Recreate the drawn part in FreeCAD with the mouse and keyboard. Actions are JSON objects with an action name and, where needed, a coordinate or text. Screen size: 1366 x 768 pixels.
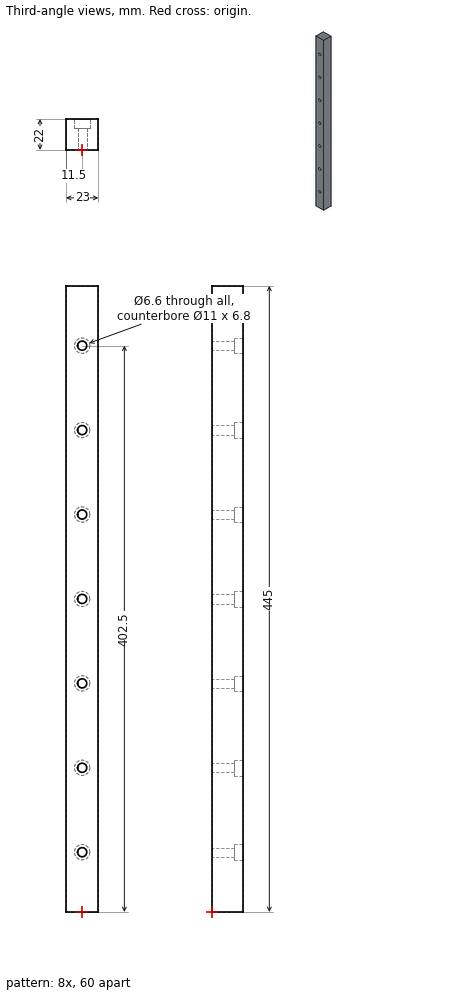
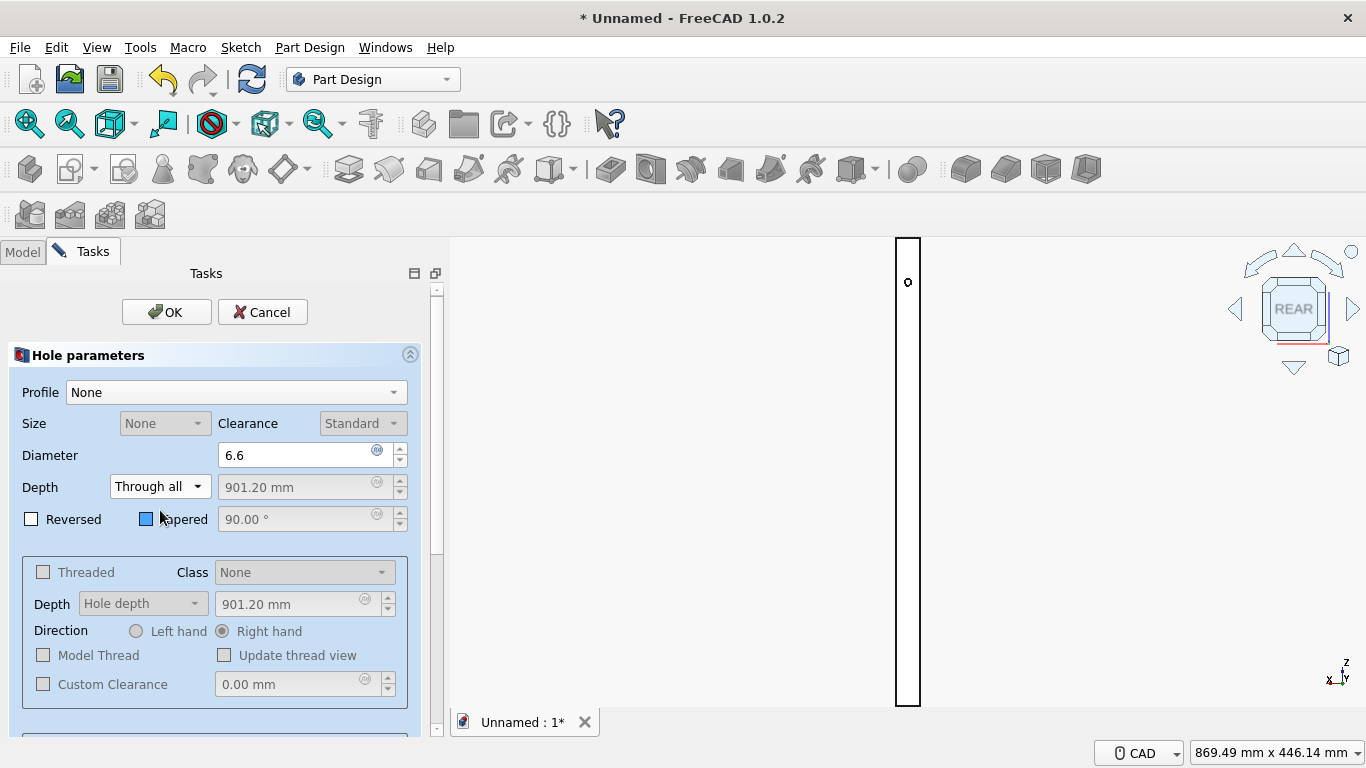
{"action": "scroll", "coordinate": [437, 510], "scroll_direction": "down", "scroll_amount": 2}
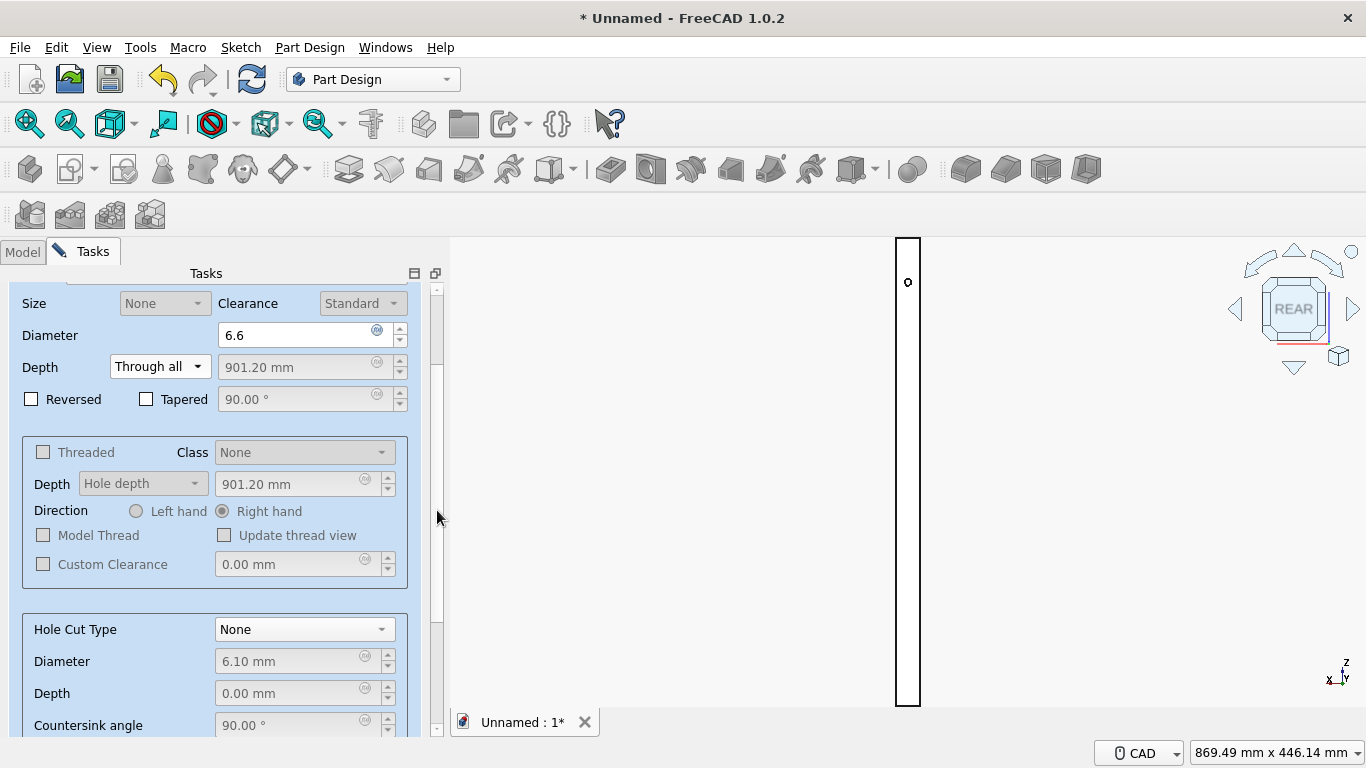
{"action": "left_click", "coordinate": [306, 630]}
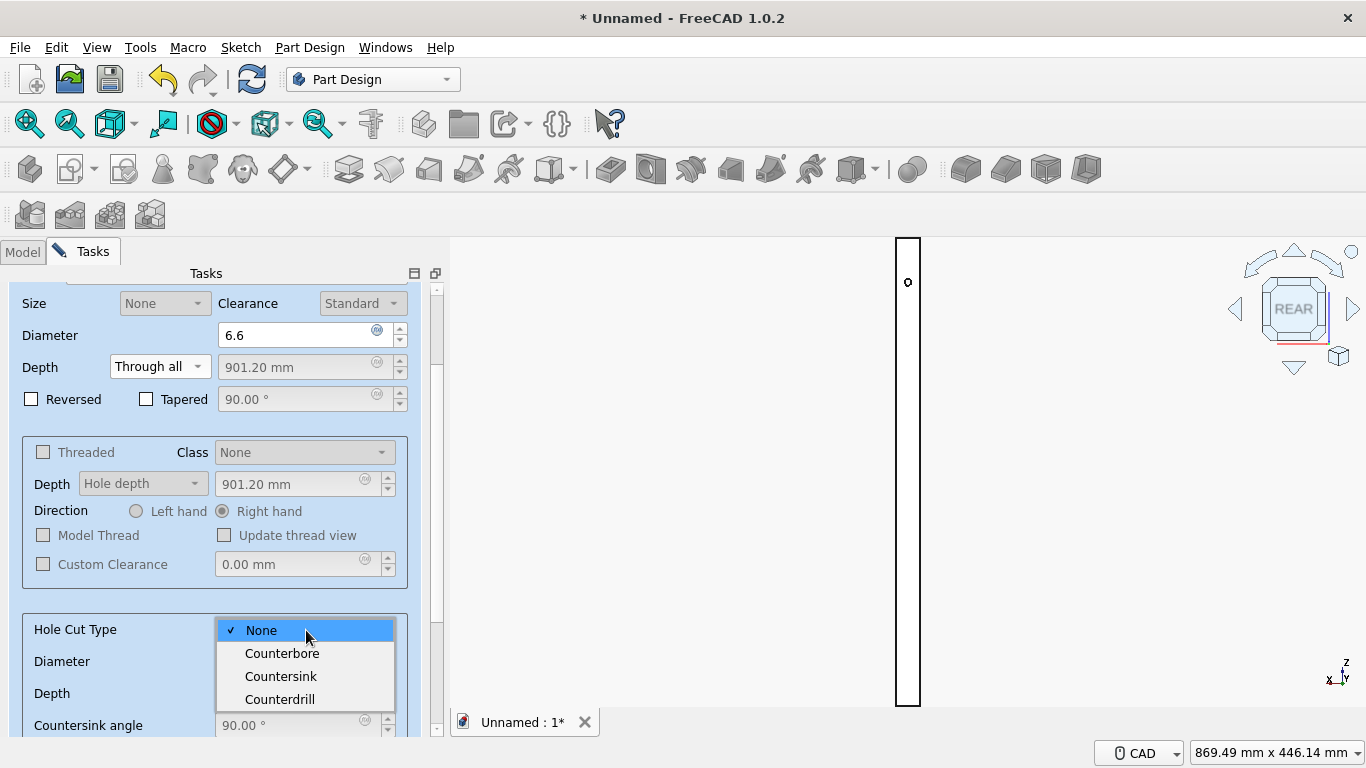
{"action": "left_click", "coordinate": [304, 654]}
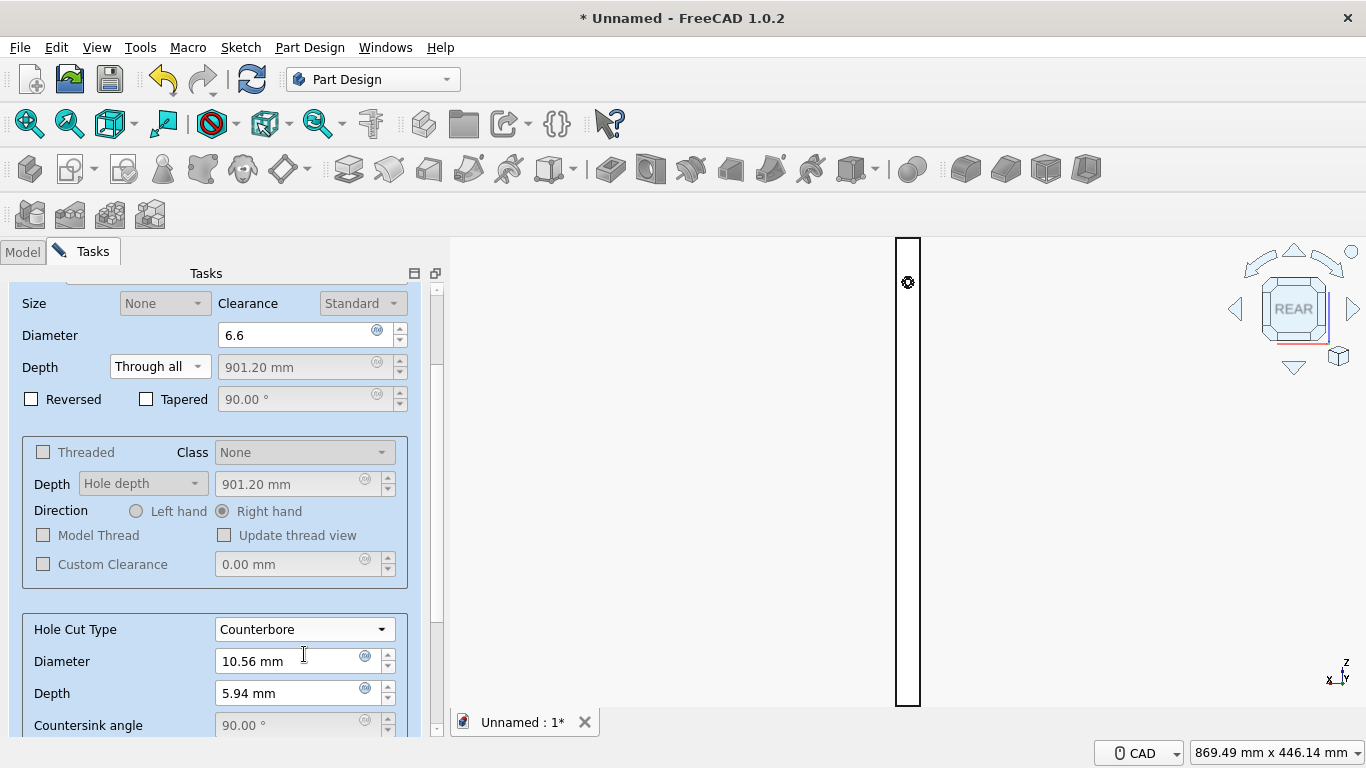
{"action": "triple_click", "coordinate": [298, 661]}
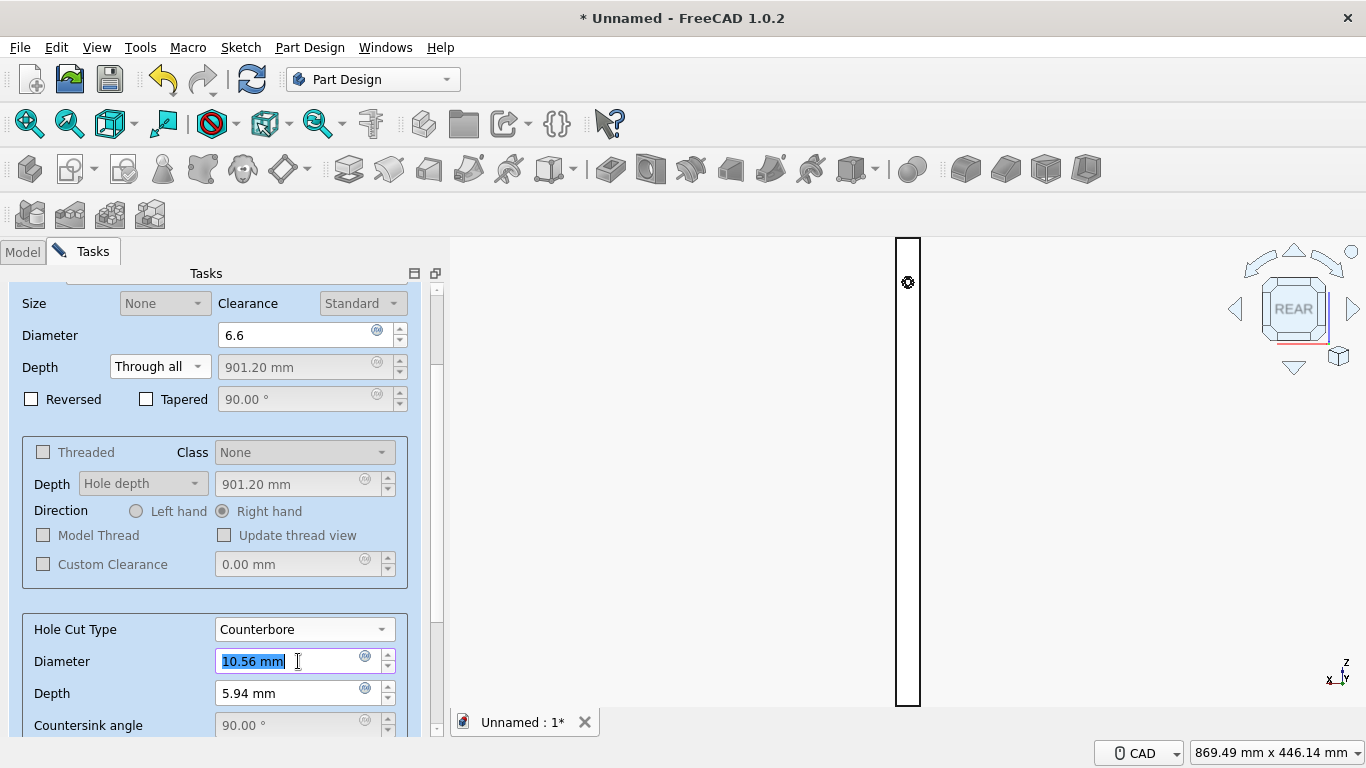
{"action": "type", "text": "11"}
{"action": "key", "text": "Tab"}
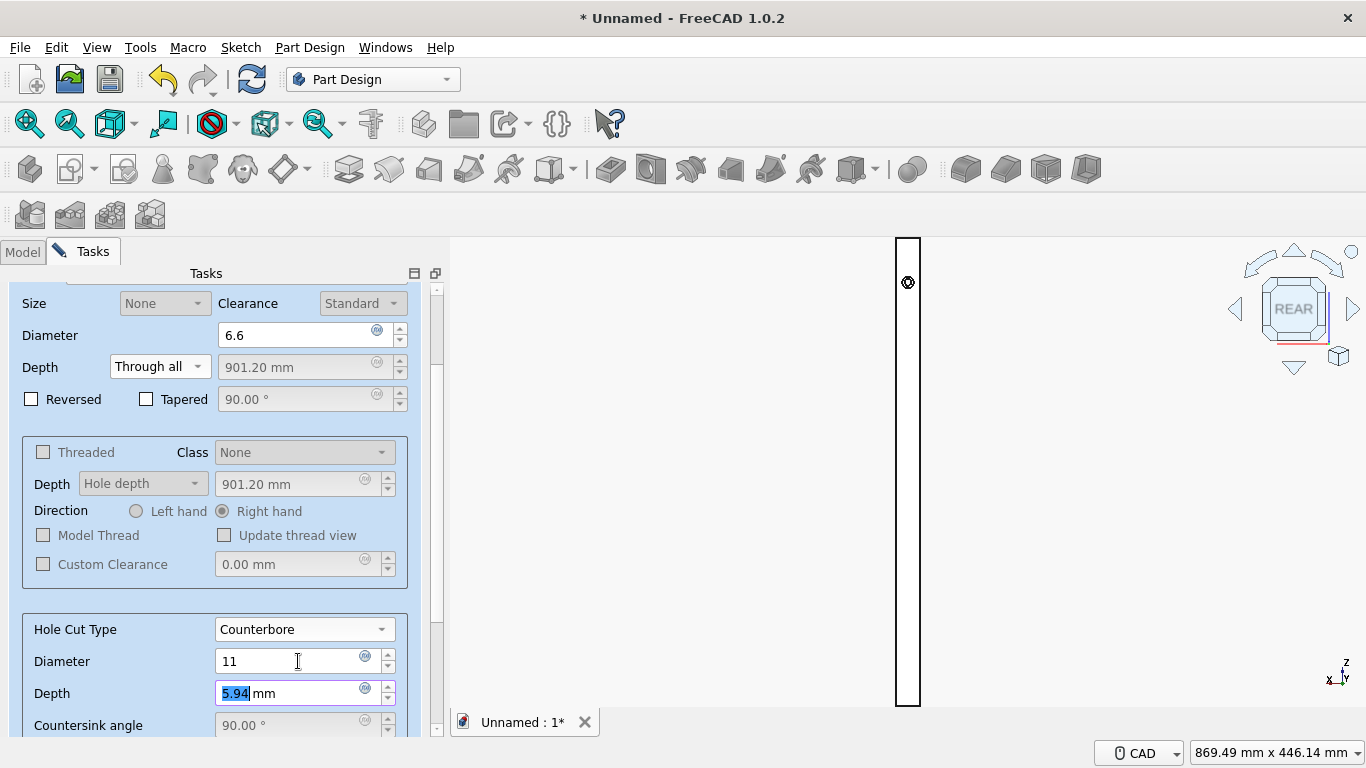
{"action": "type", "text": "6.8"}
{"action": "key", "text": "Tab"}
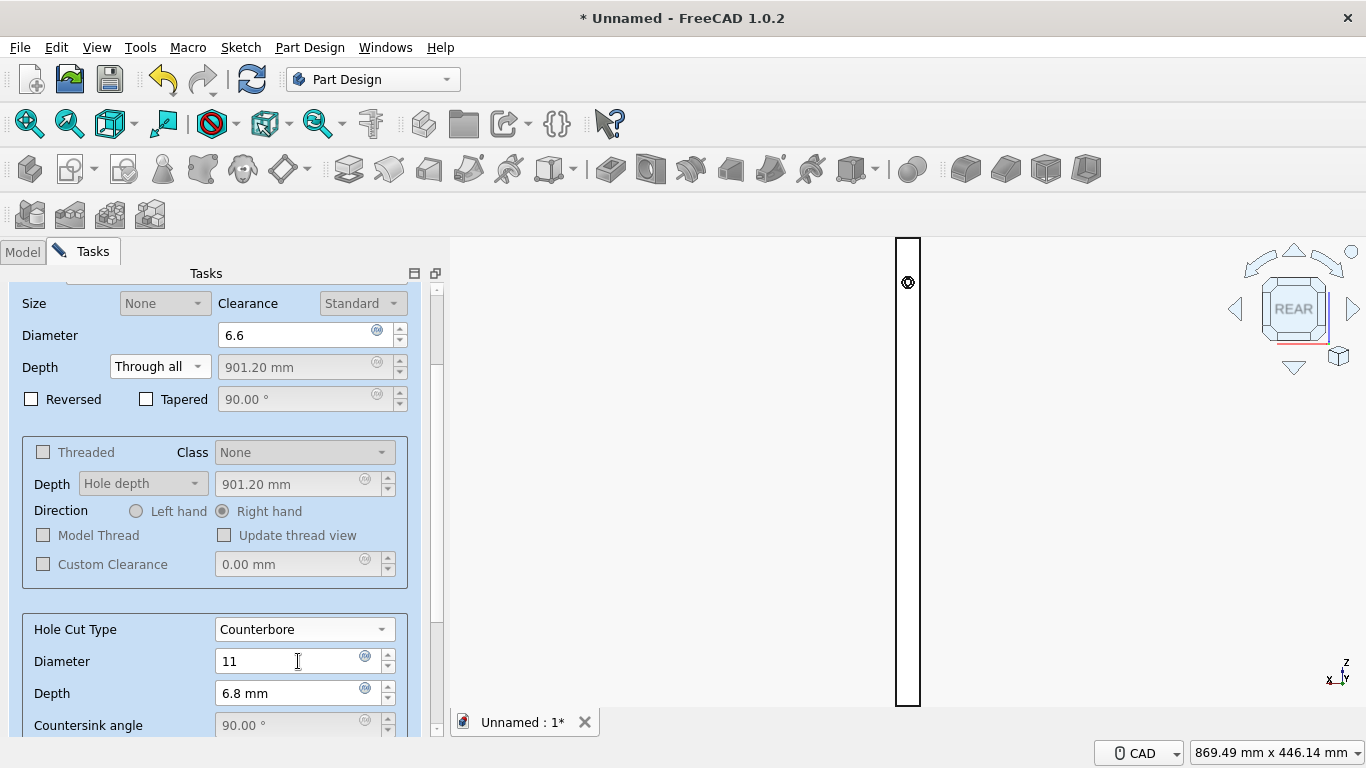
{"action": "scroll", "coordinate": [437, 510], "scroll_direction": "up", "scroll_amount": 3}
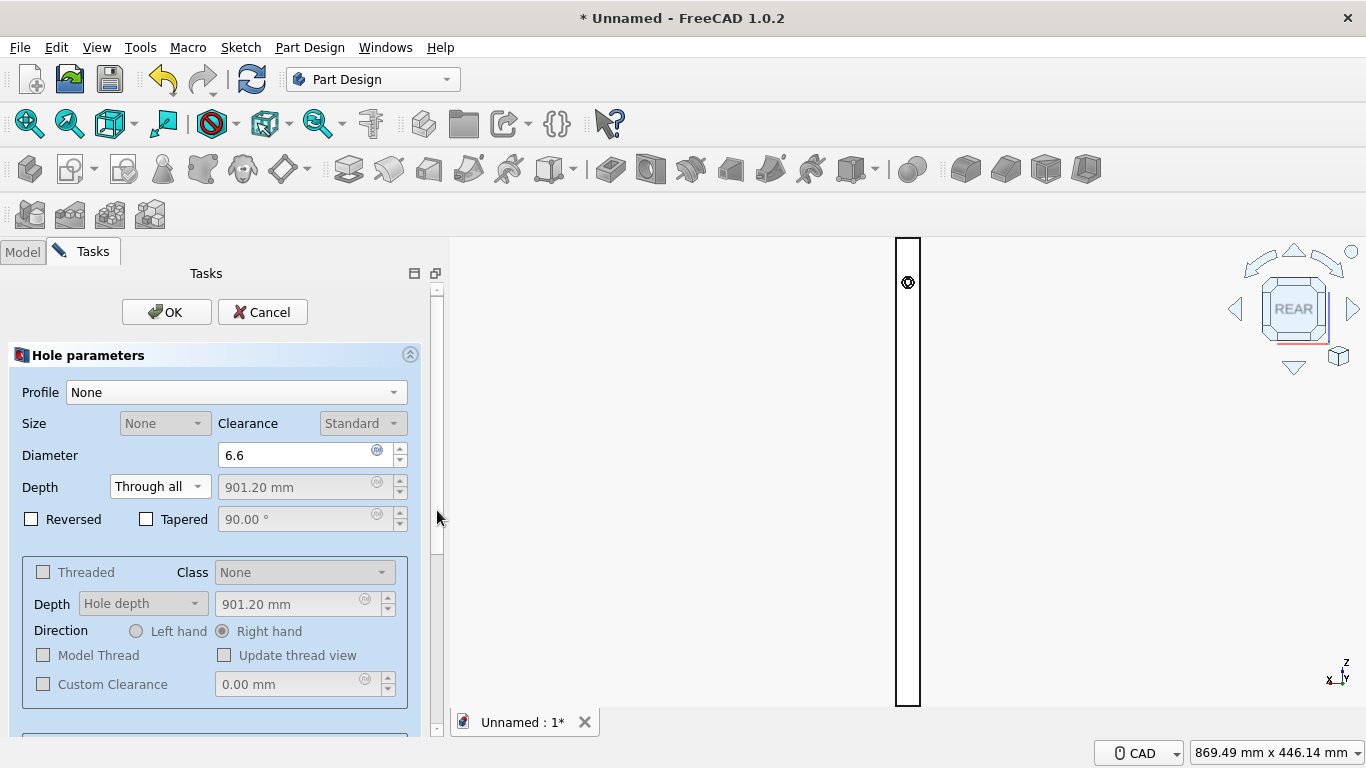
{"action": "left_click", "coordinate": [167, 312]}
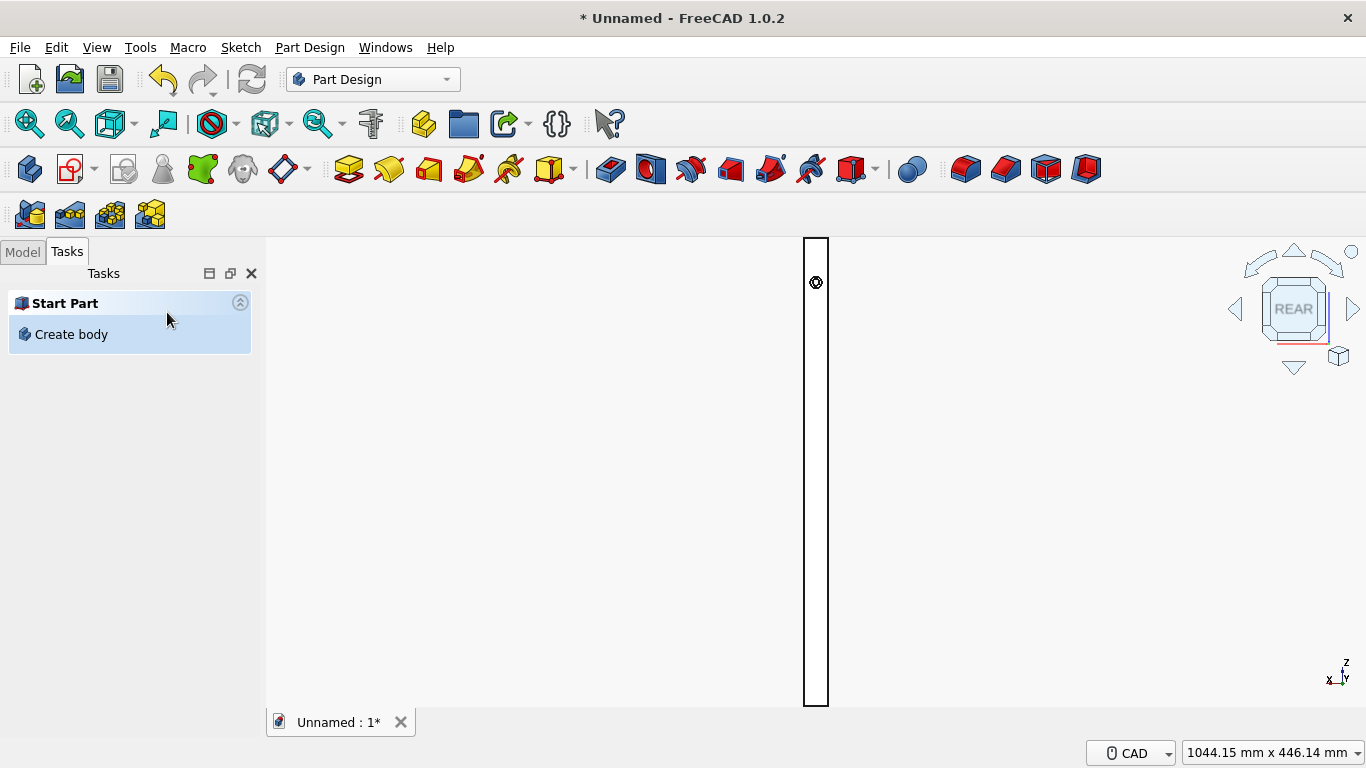
{"action": "left_click", "coordinate": [23, 251]}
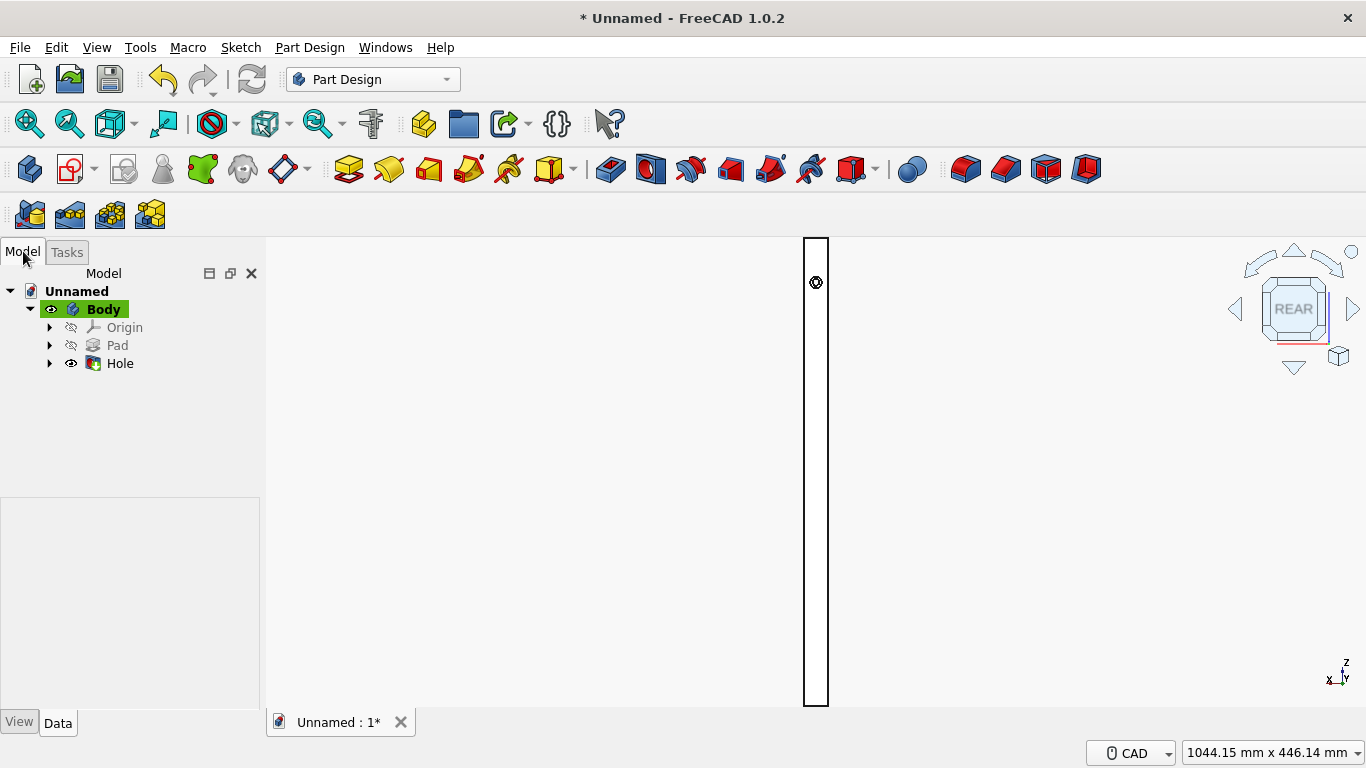
{"action": "left_click", "coordinate": [116, 363]}